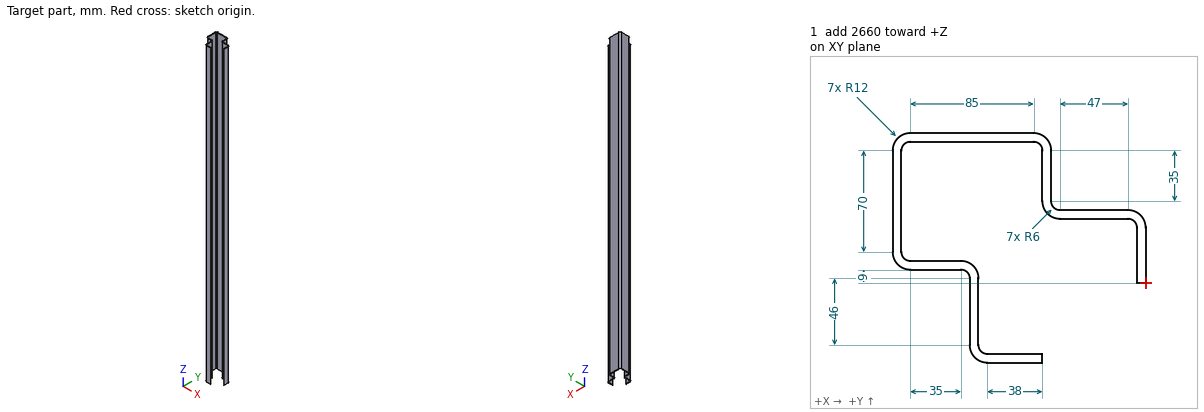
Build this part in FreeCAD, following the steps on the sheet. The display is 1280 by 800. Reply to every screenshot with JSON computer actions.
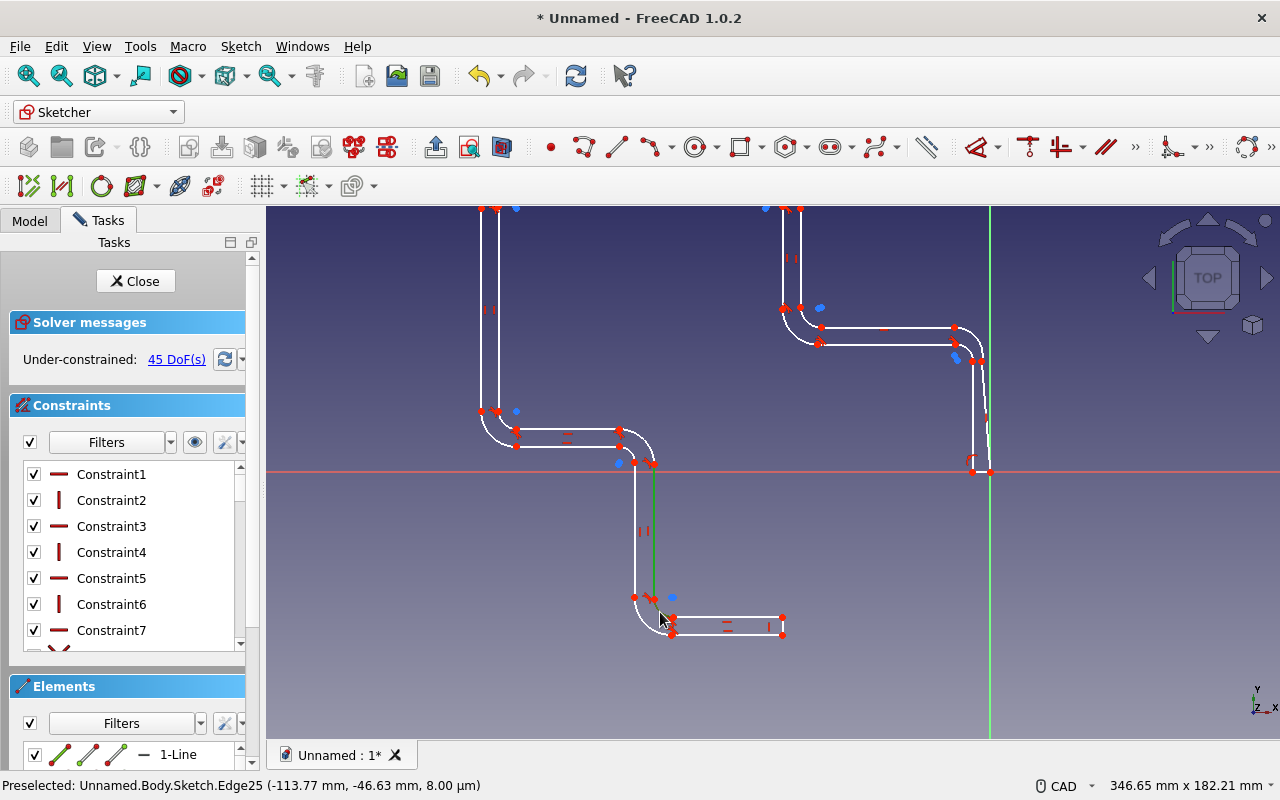
{"action": "key", "text": "t"}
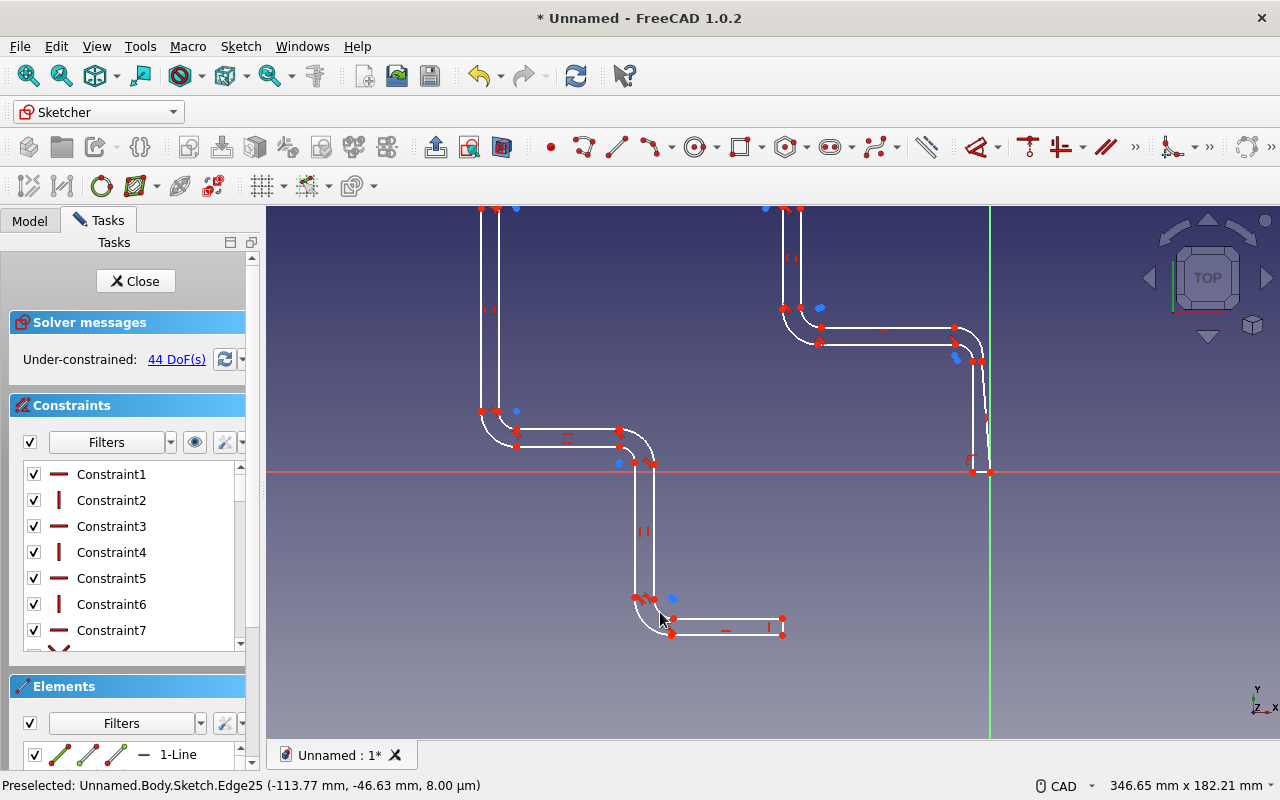
{"action": "left_click", "coordinate": [654, 559]}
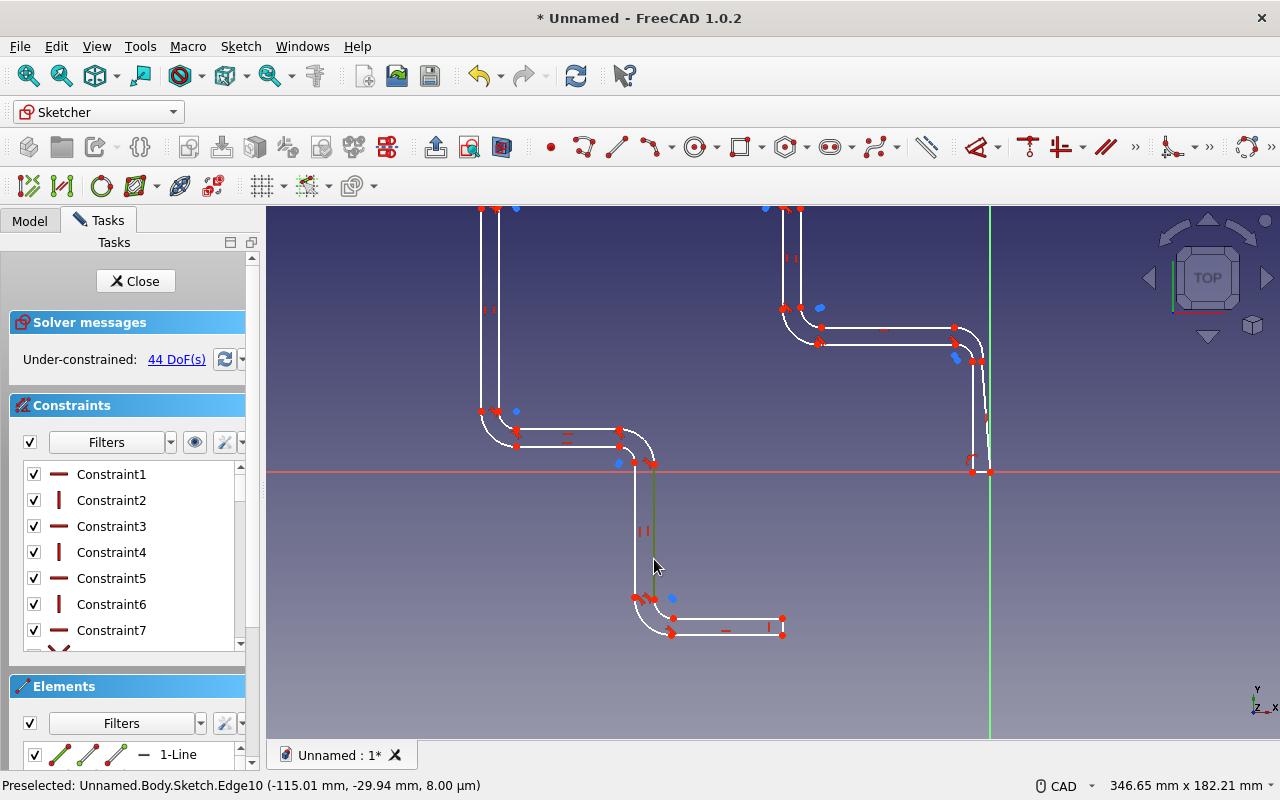
{"action": "left_click", "coordinate": [650, 448]}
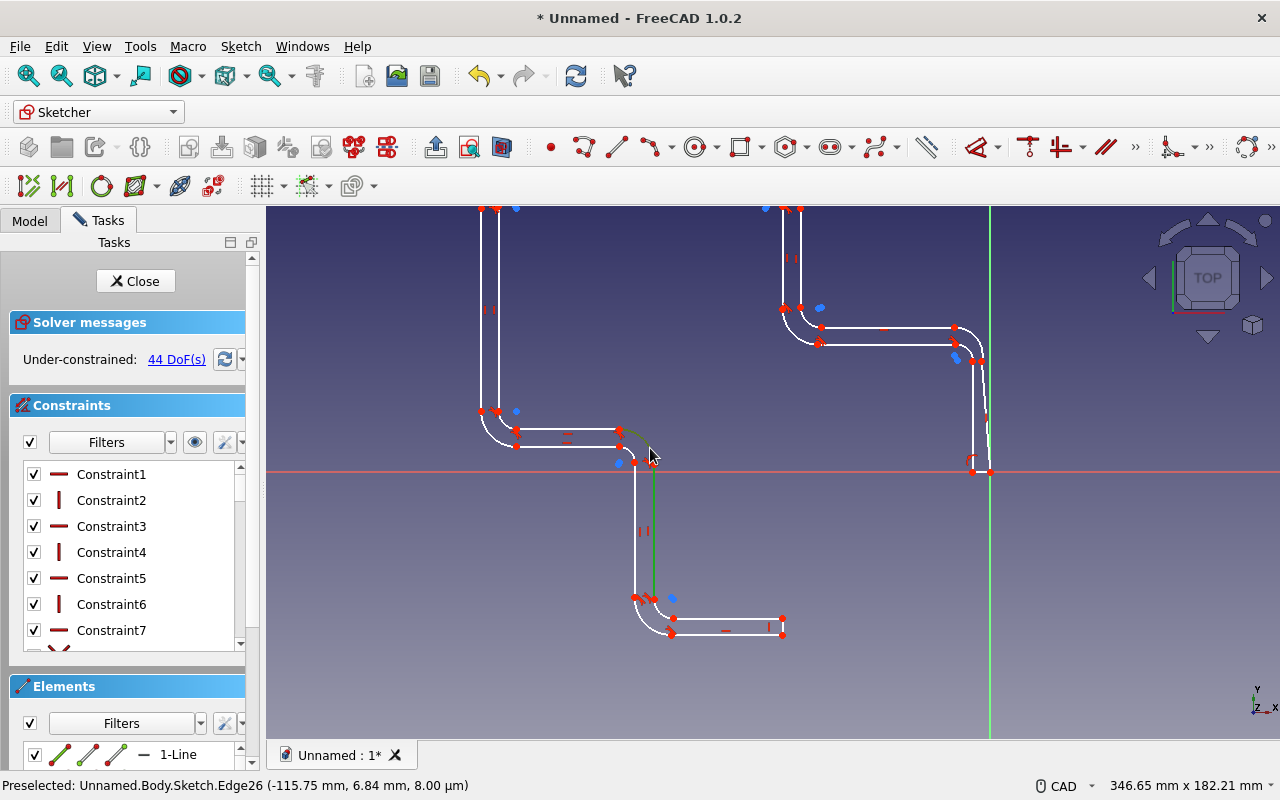
{"action": "key", "text": "t"}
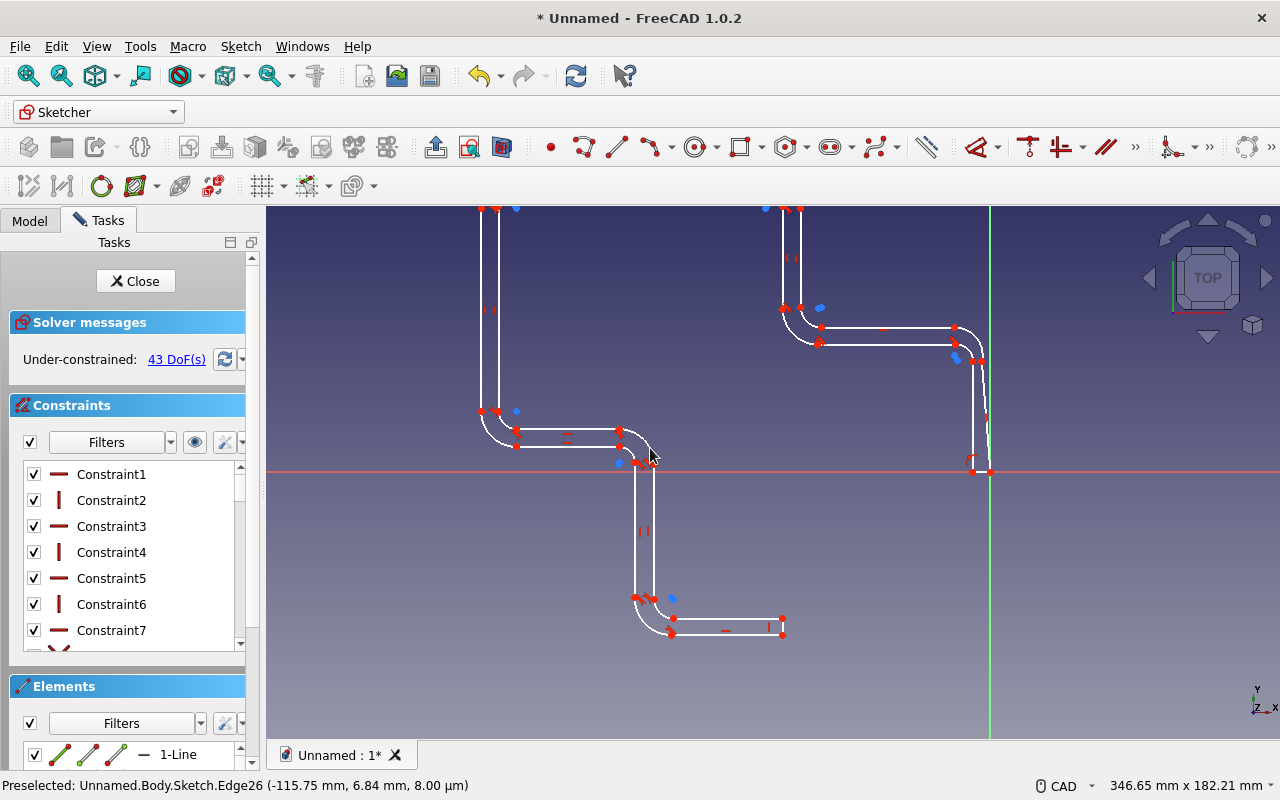
{"action": "left_click", "coordinate": [588, 429]}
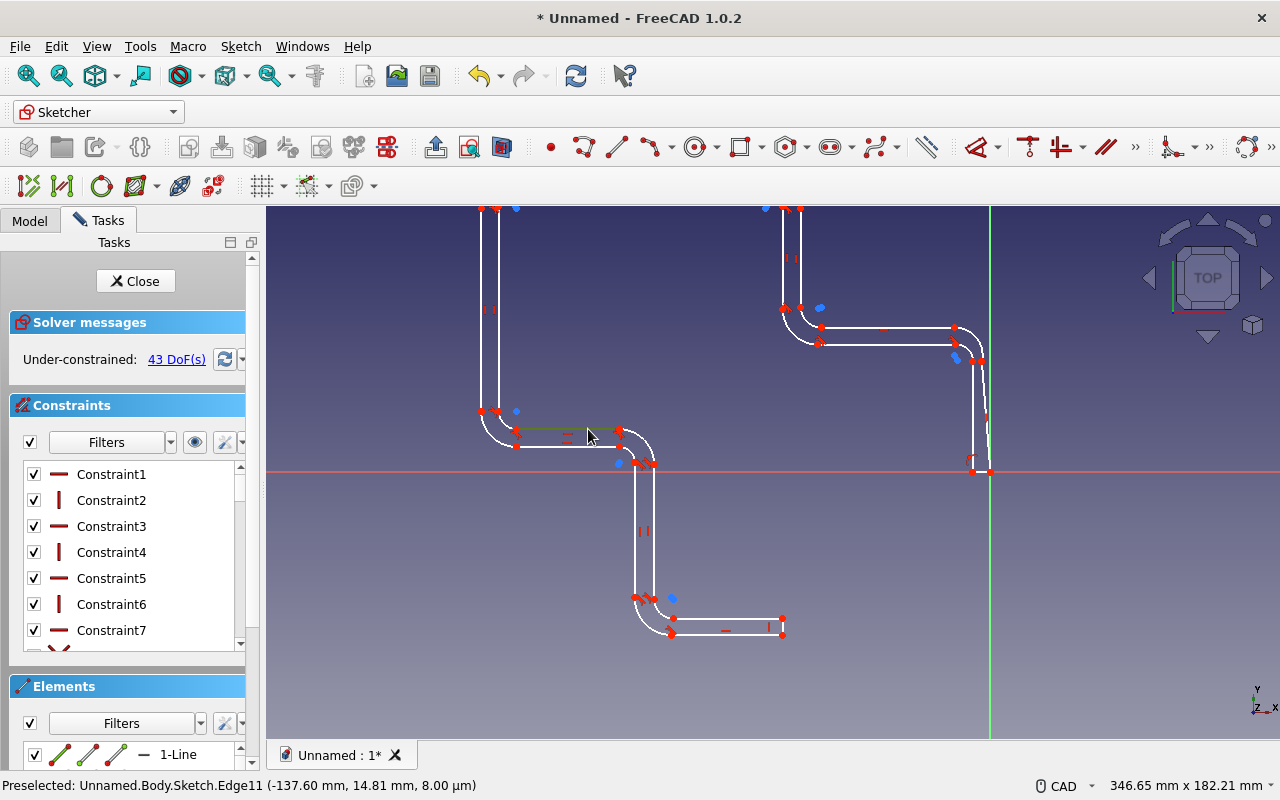
{"action": "left_click", "coordinate": [650, 449]}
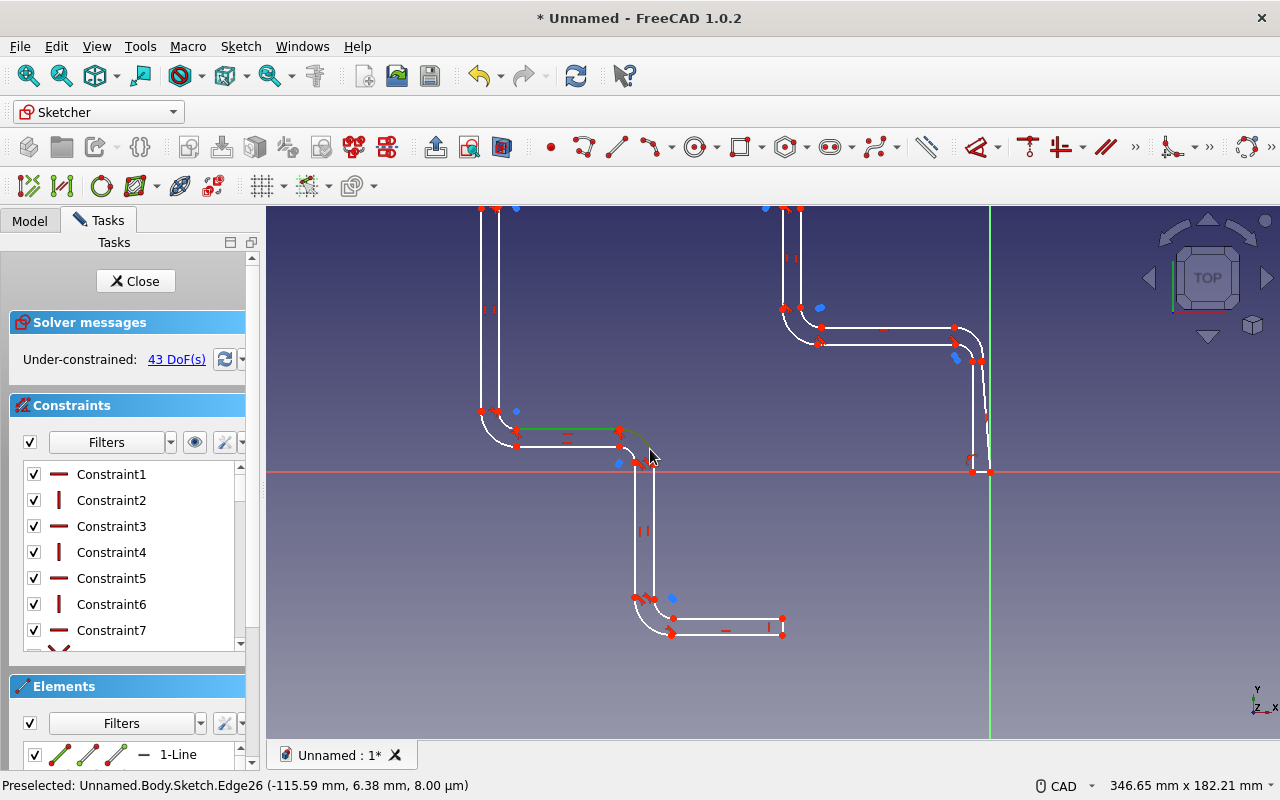
{"action": "key", "text": "t"}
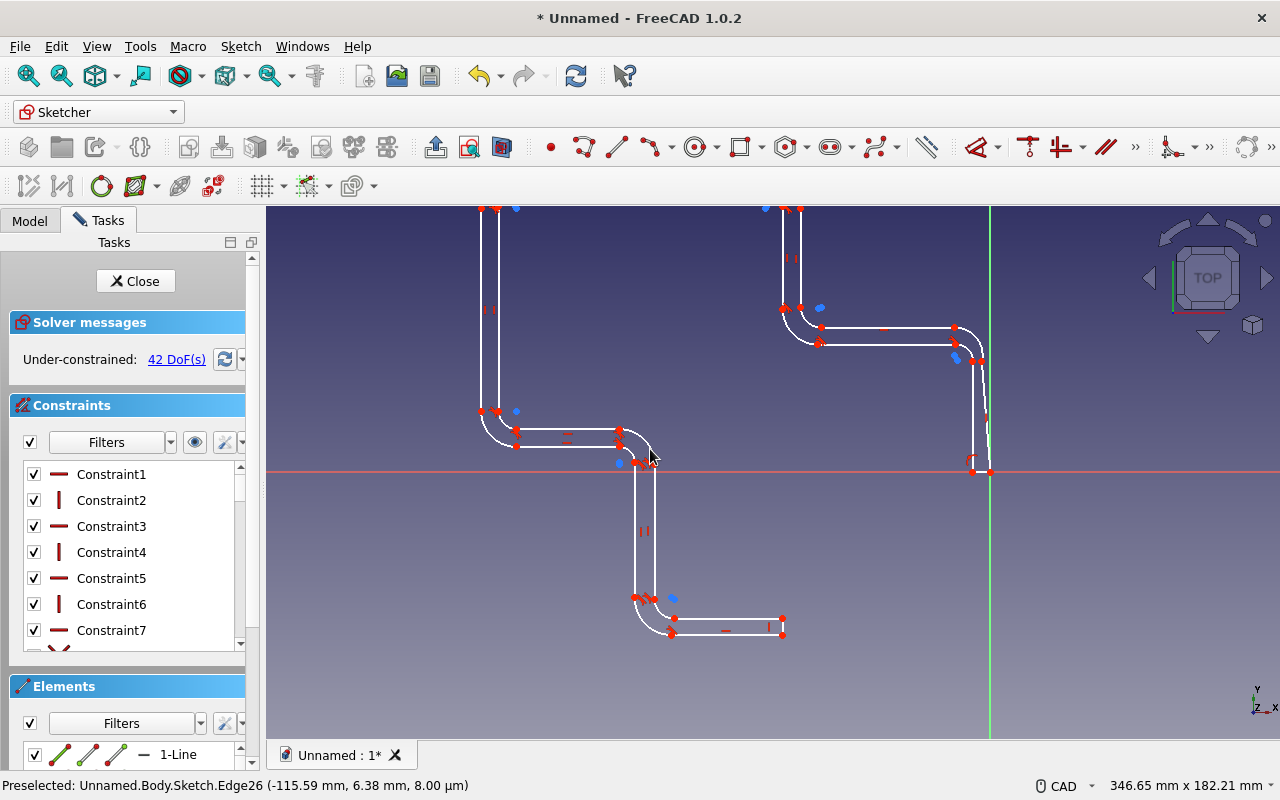
{"action": "left_click", "coordinate": [588, 429]}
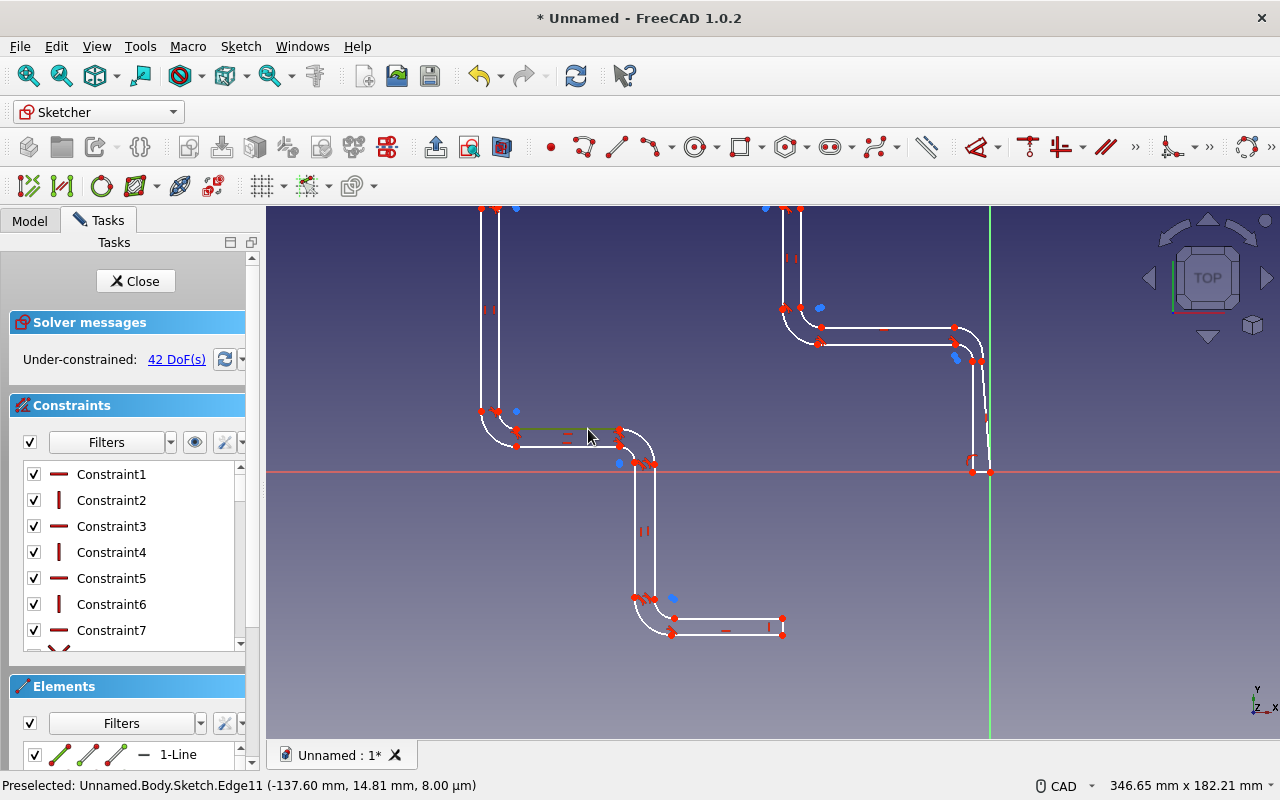
{"action": "left_click", "coordinate": [504, 424]}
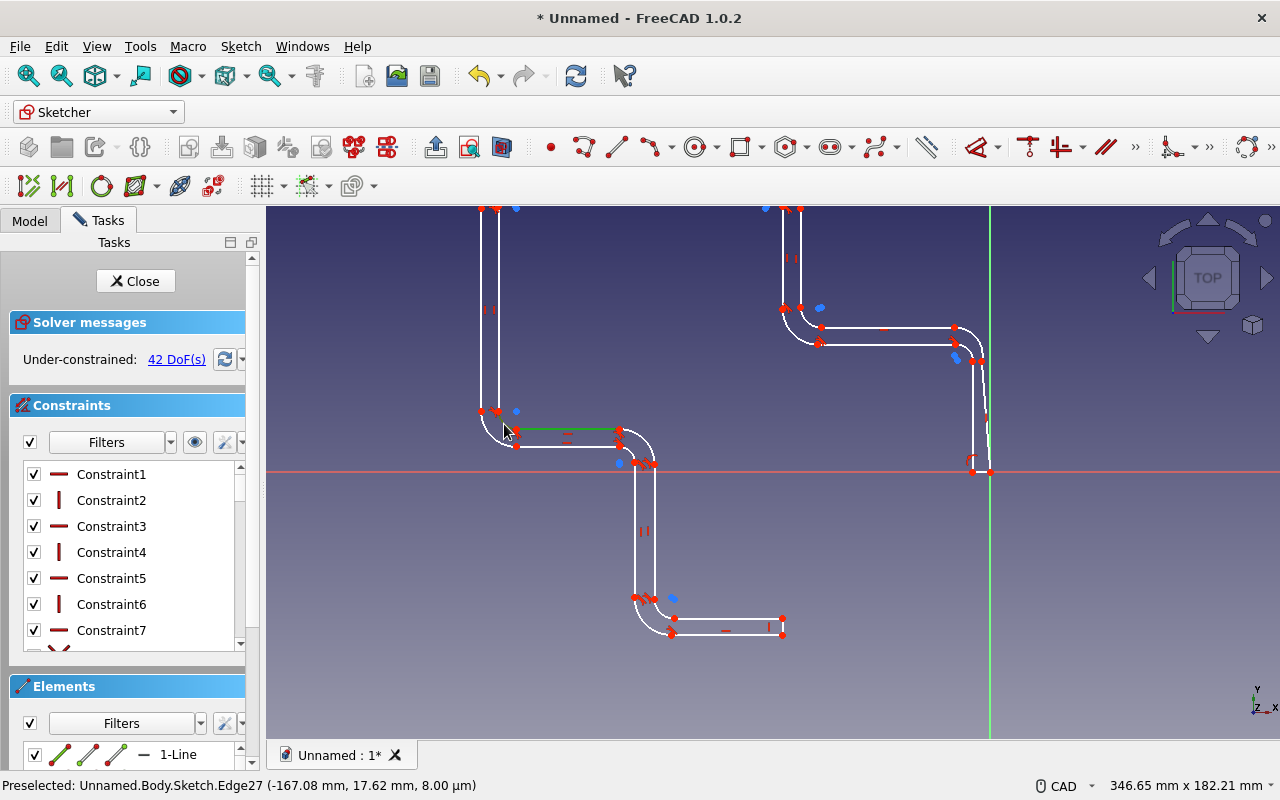
{"action": "key", "text": "t"}